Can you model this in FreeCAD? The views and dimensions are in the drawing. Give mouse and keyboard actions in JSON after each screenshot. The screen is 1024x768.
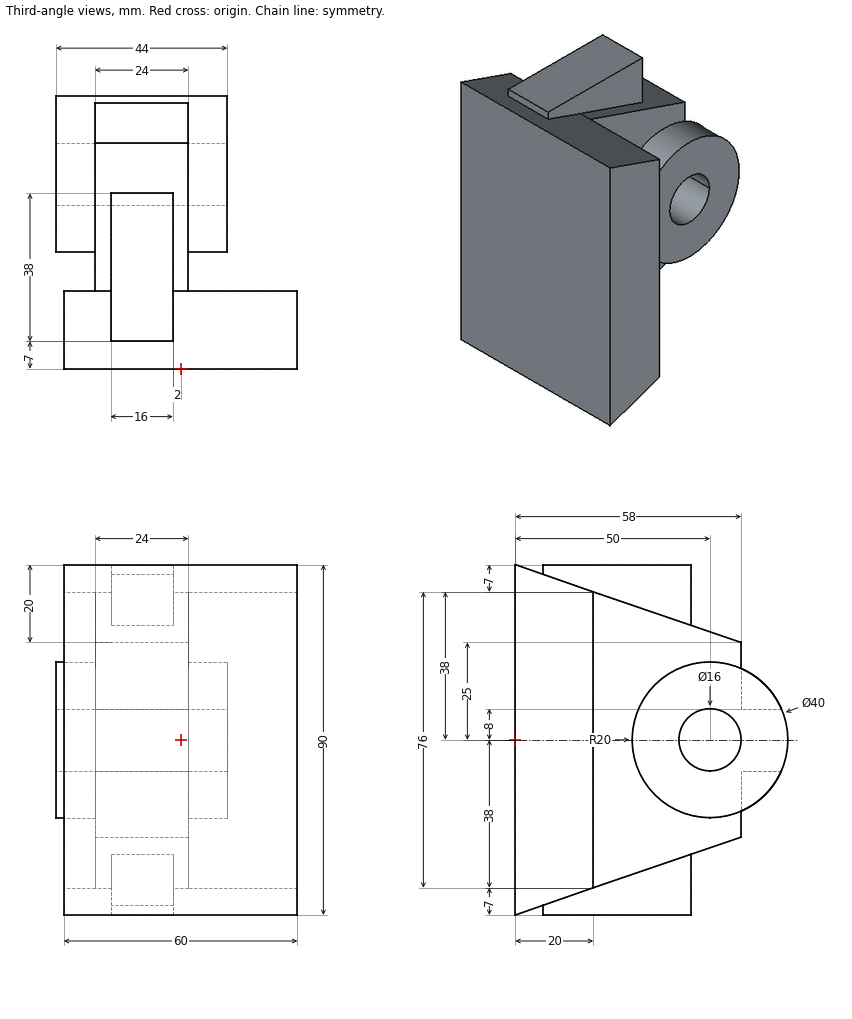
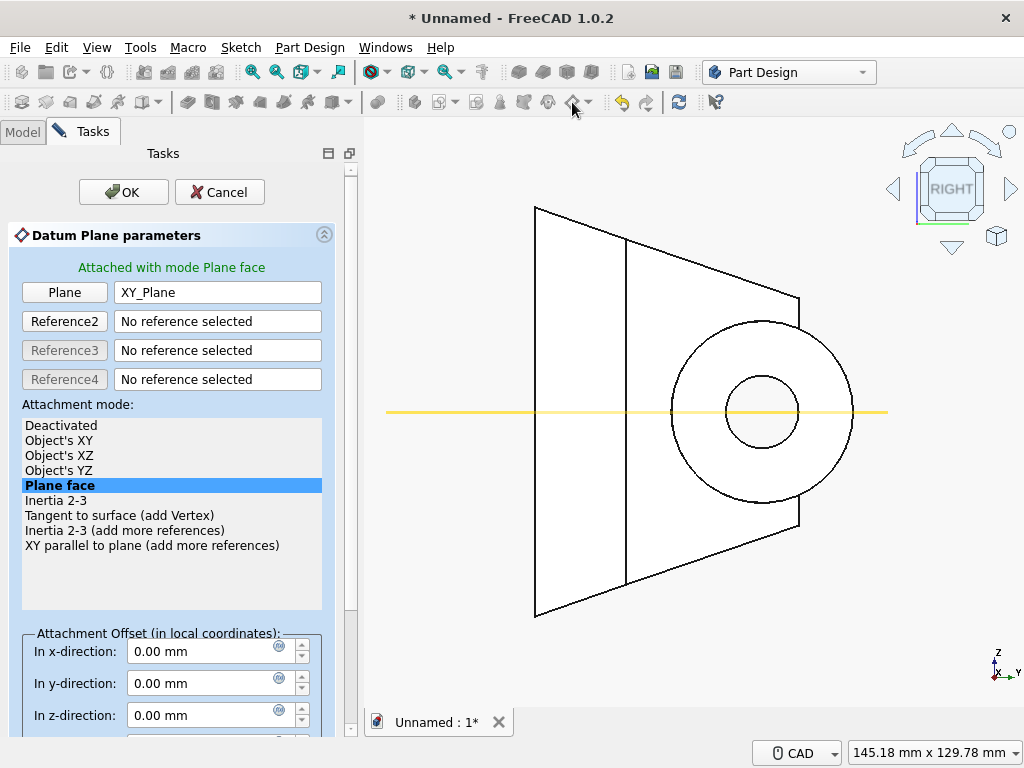
{"action": "triple_click", "coordinate": [210, 715]}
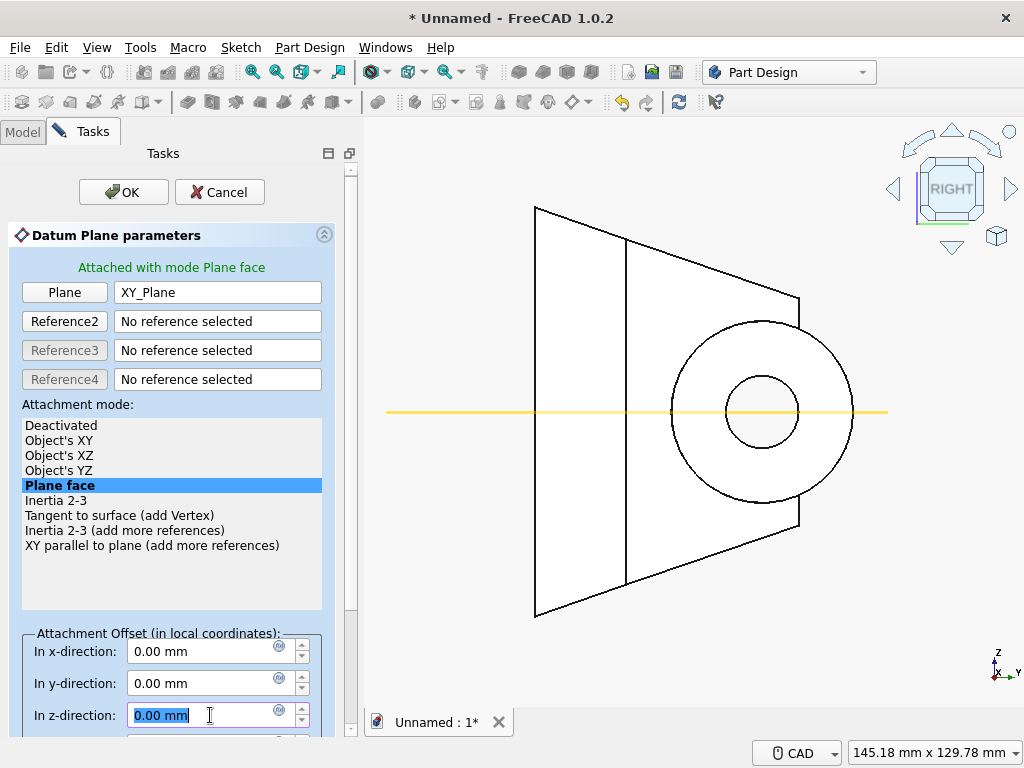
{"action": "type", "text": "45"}
{"action": "key", "text": "Tab"}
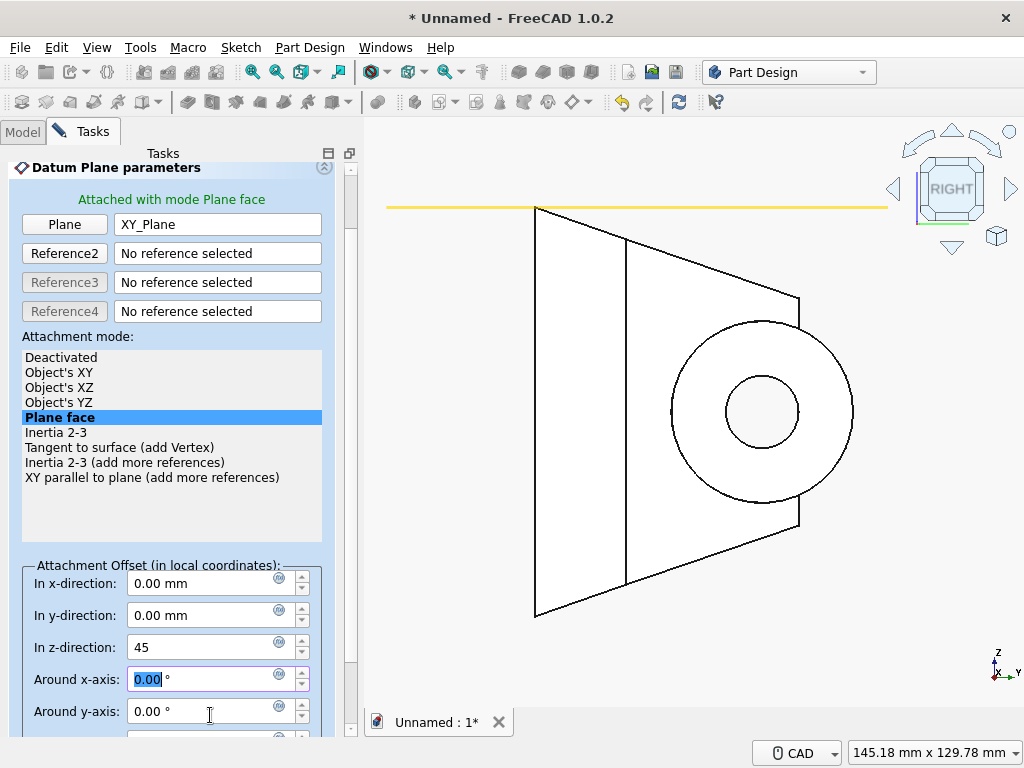
{"action": "scroll", "coordinate": [351, 450], "scroll_direction": "up", "scroll_amount": 2}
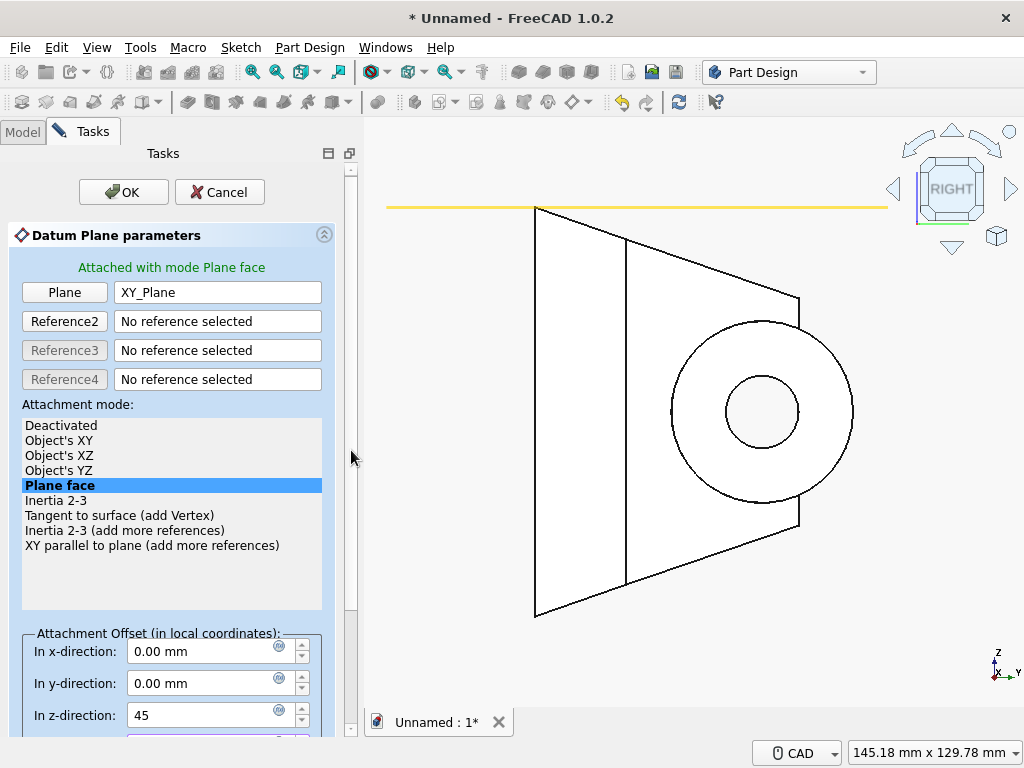
{"action": "left_click", "coordinate": [124, 192]}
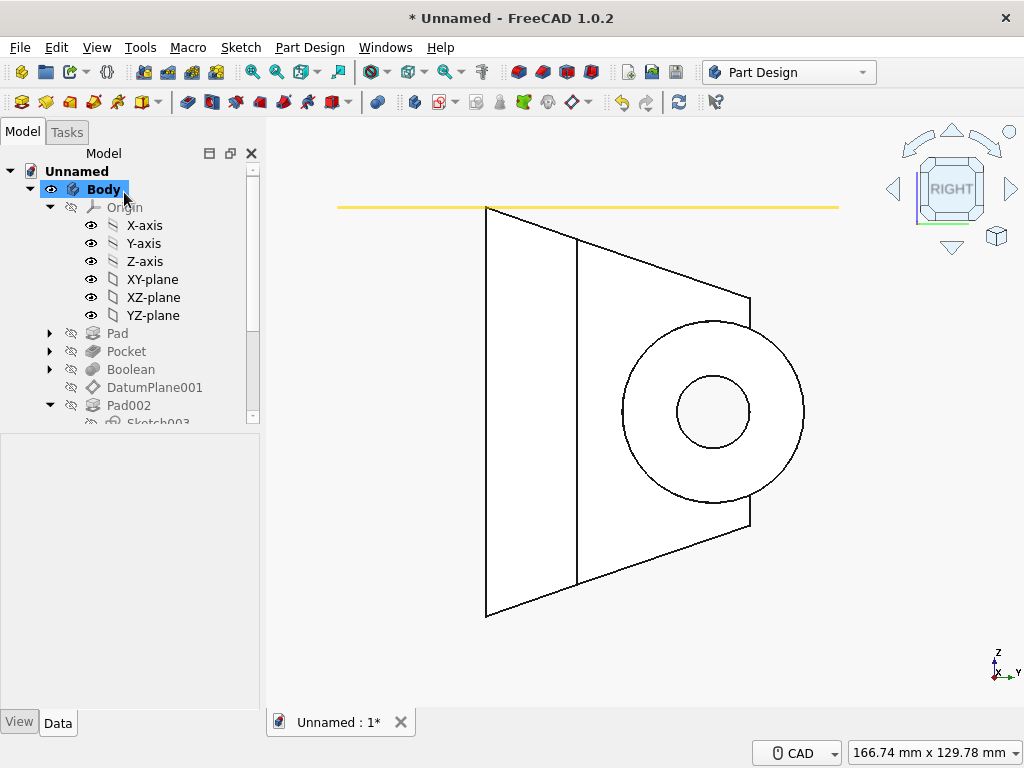
{"action": "scroll", "coordinate": [100, 293], "scroll_direction": "down", "scroll_amount": 3}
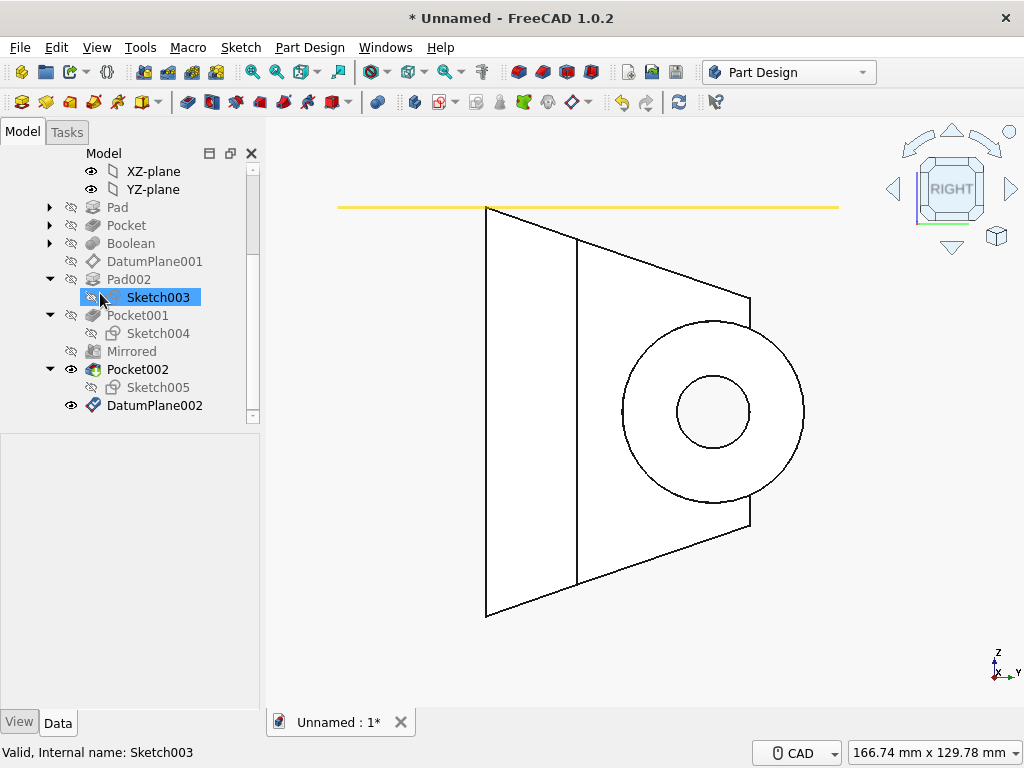
{"action": "left_click", "coordinate": [116, 405]}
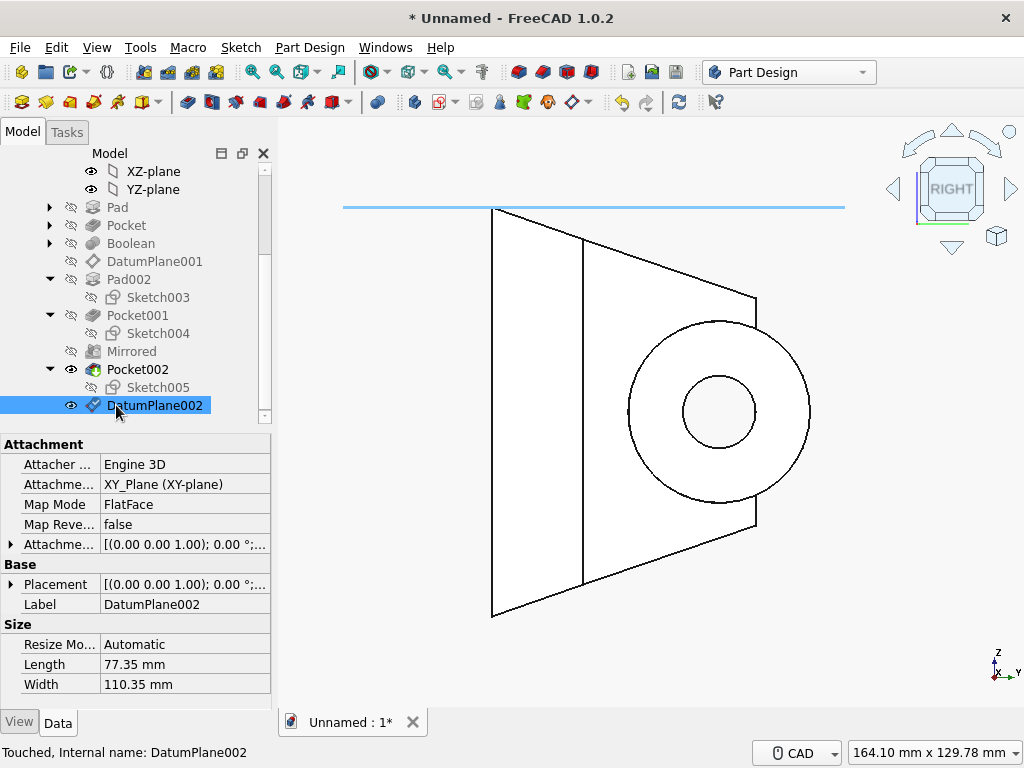
{"action": "left_click", "coordinate": [440, 102]}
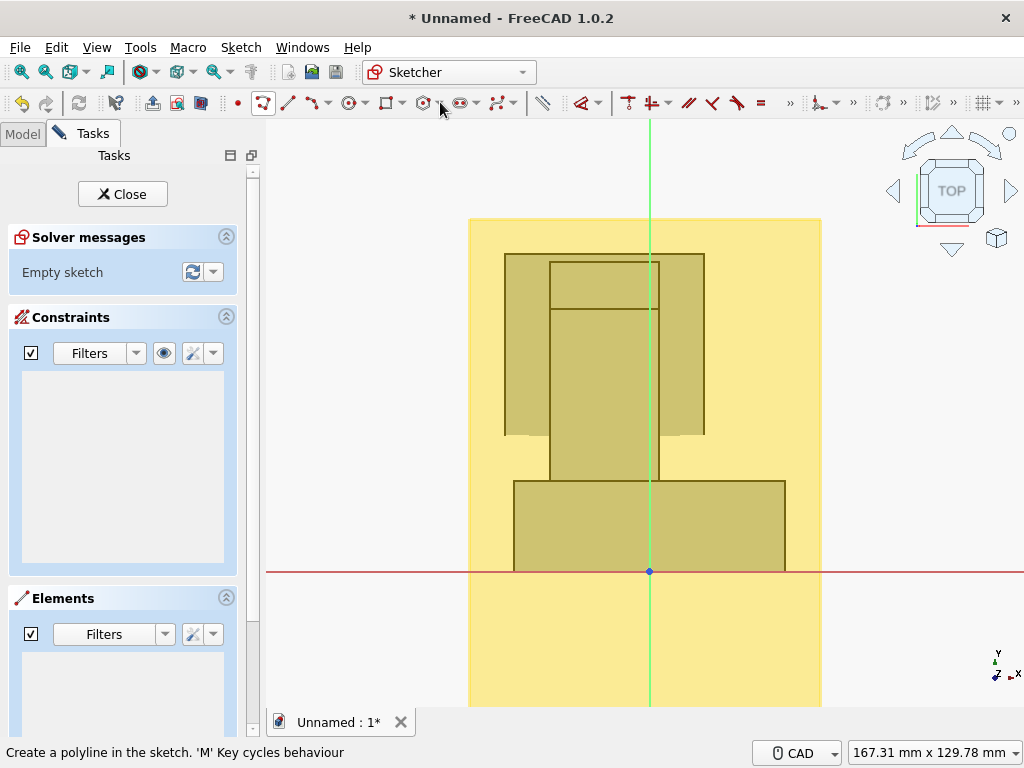
{"action": "scroll", "coordinate": [648, 539], "scroll_direction": "up", "scroll_amount": 3}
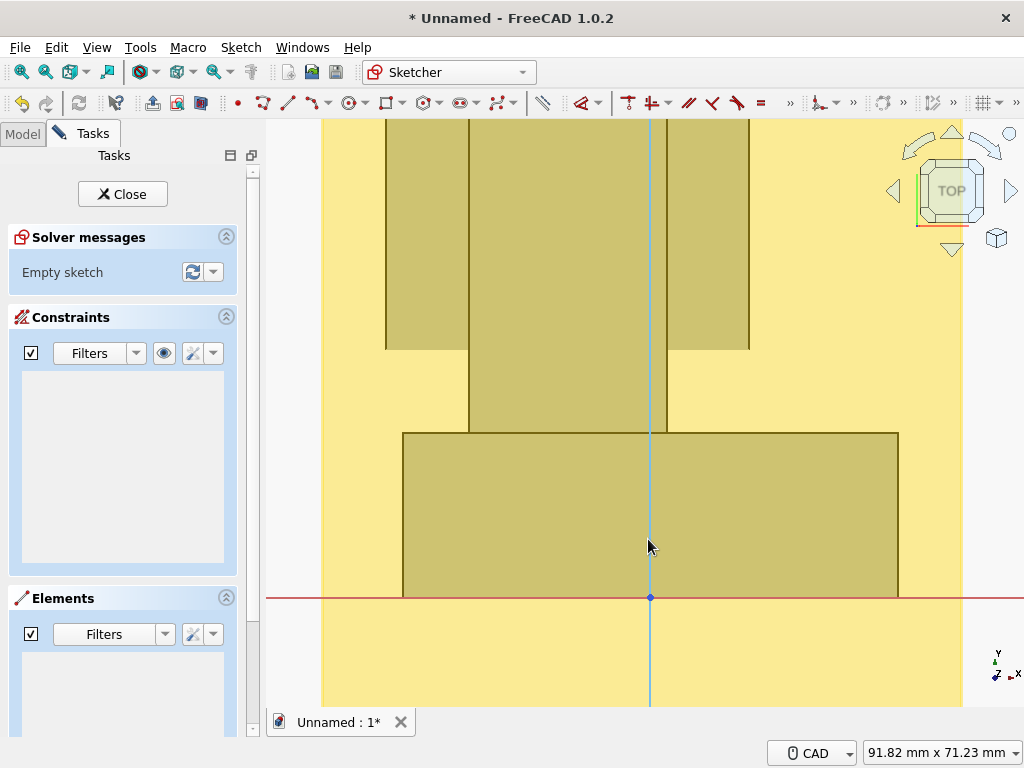
{"action": "left_click", "coordinate": [386, 104]}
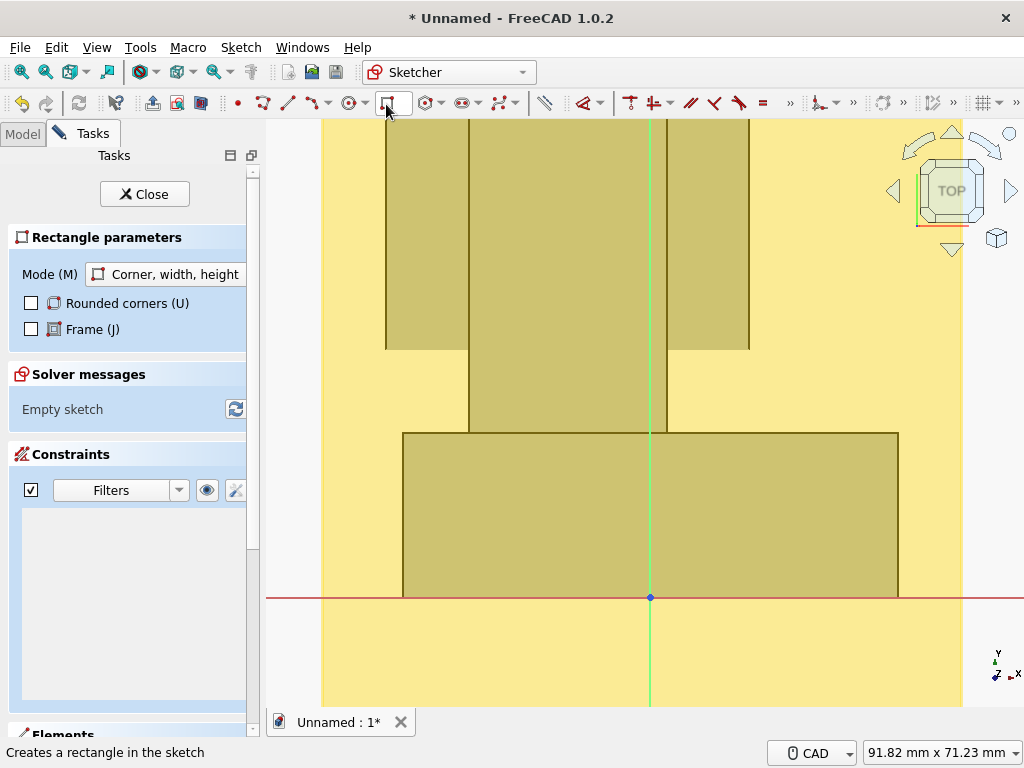
{"action": "left_click", "coordinate": [502, 226]}
{"action": "mouse_move", "coordinate": [634, 540]}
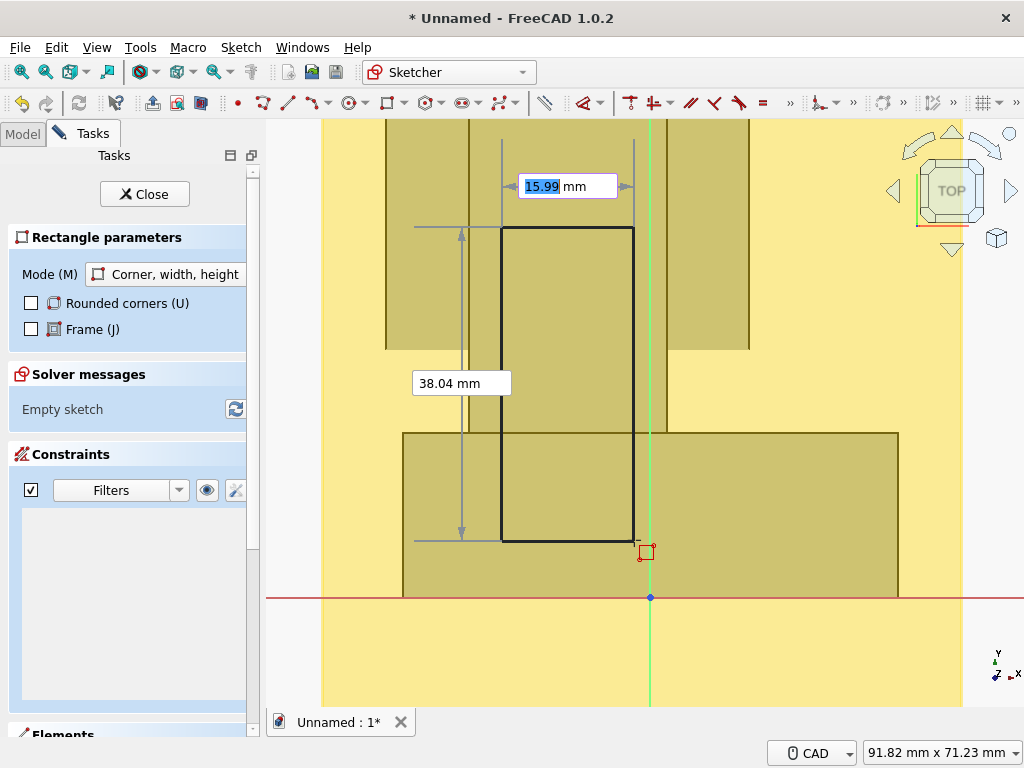
{"action": "type", "text": "16"}
{"action": "key", "text": "Tab"}
{"action": "type", "text": "38"}
{"action": "key", "text": "Return"}
{"action": "key", "text": "Escape"}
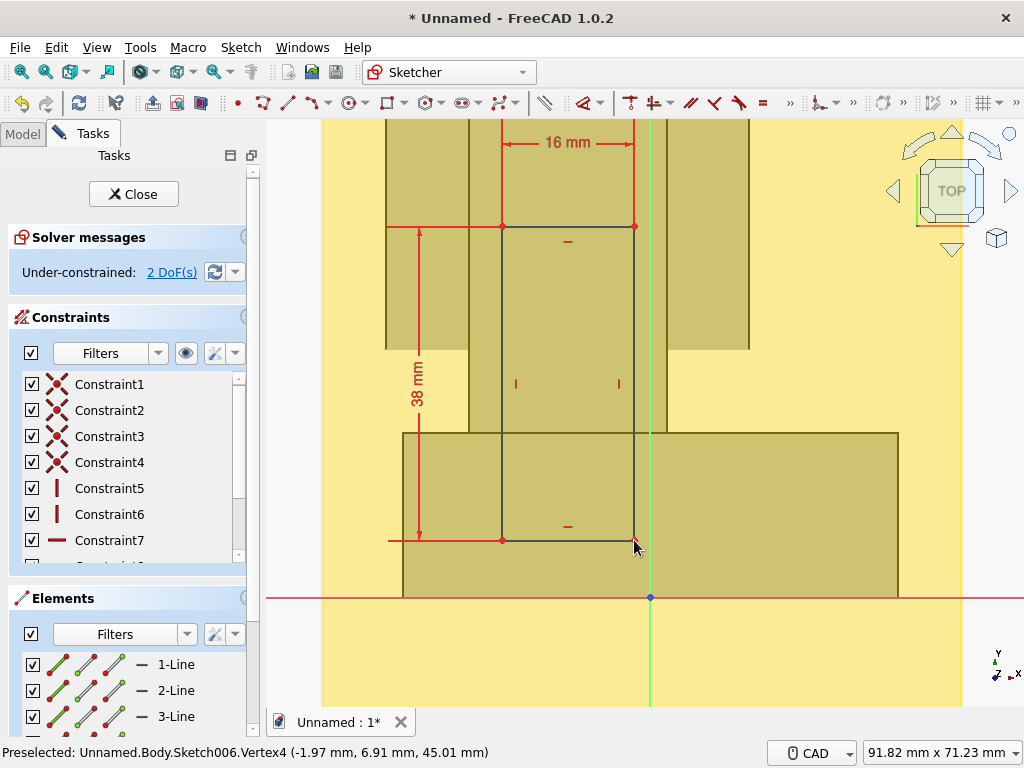
{"action": "left_click", "coordinate": [584, 104]}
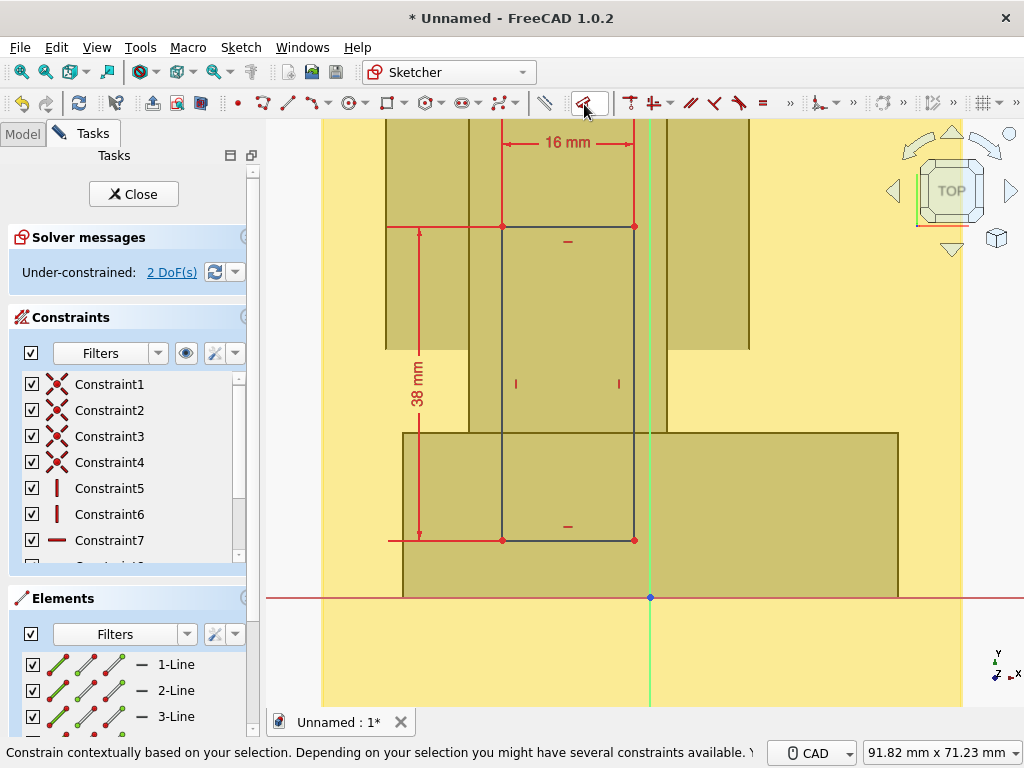
{"action": "left_click", "coordinate": [502, 541]}
{"action": "left_click", "coordinate": [684, 569]}